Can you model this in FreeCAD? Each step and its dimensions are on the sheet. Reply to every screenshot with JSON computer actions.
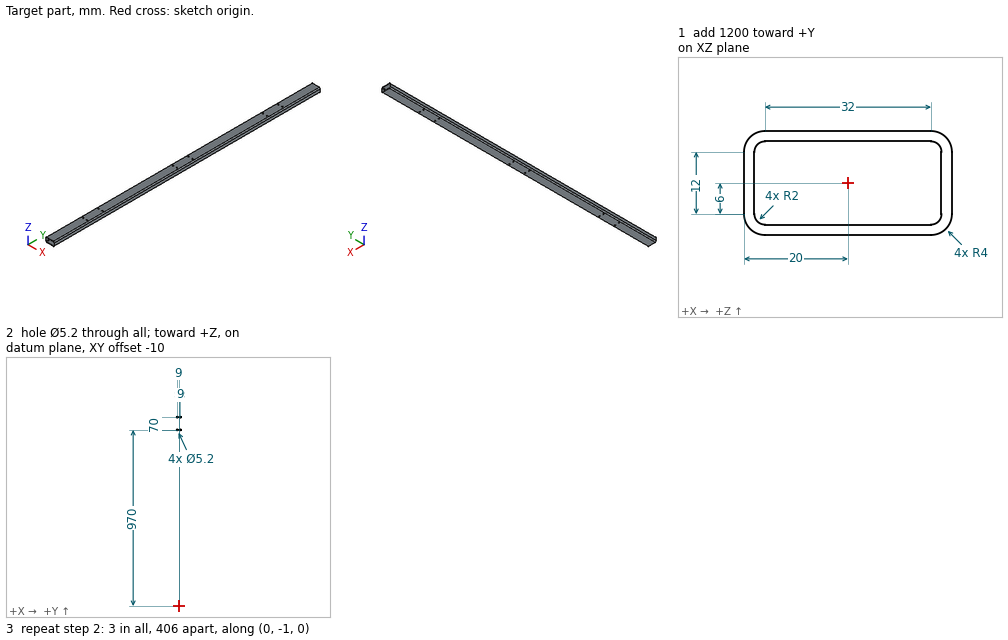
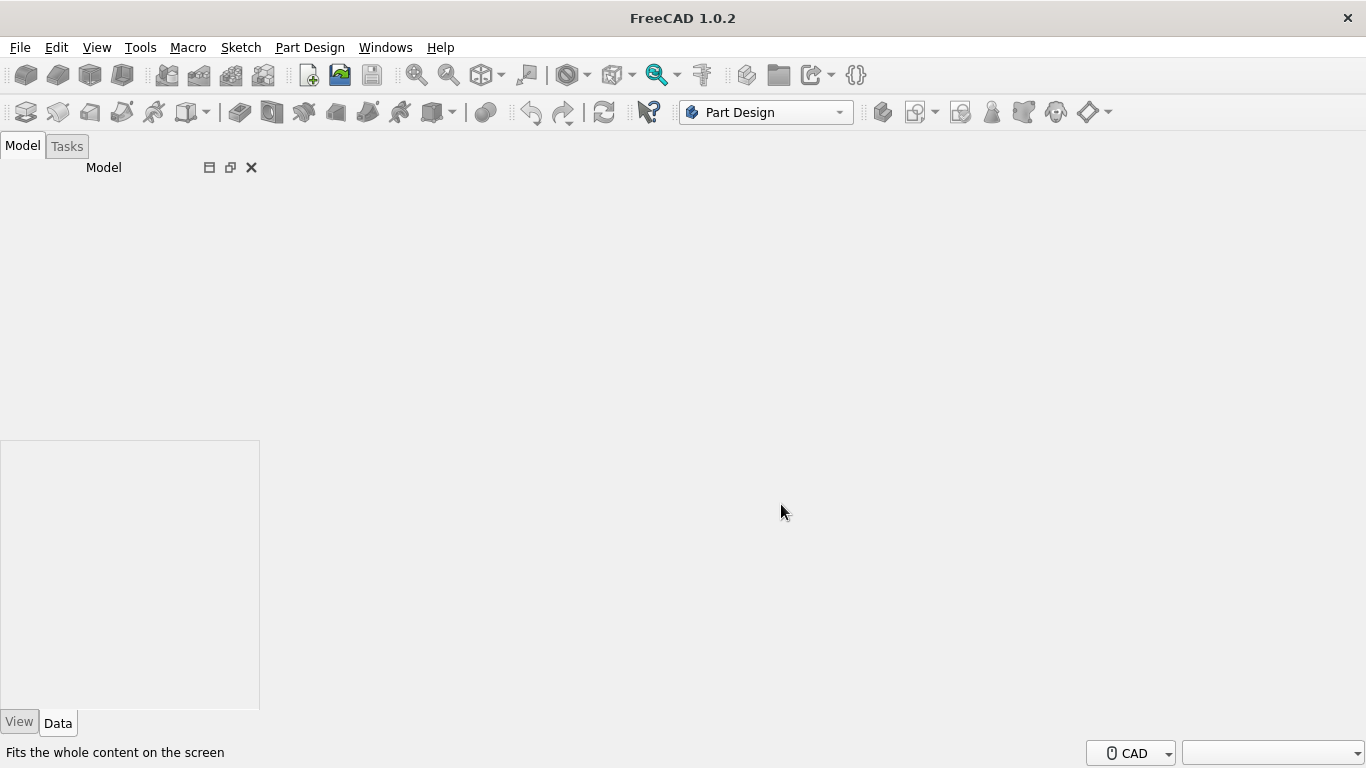
{"action": "left_click", "coordinate": [308, 76]}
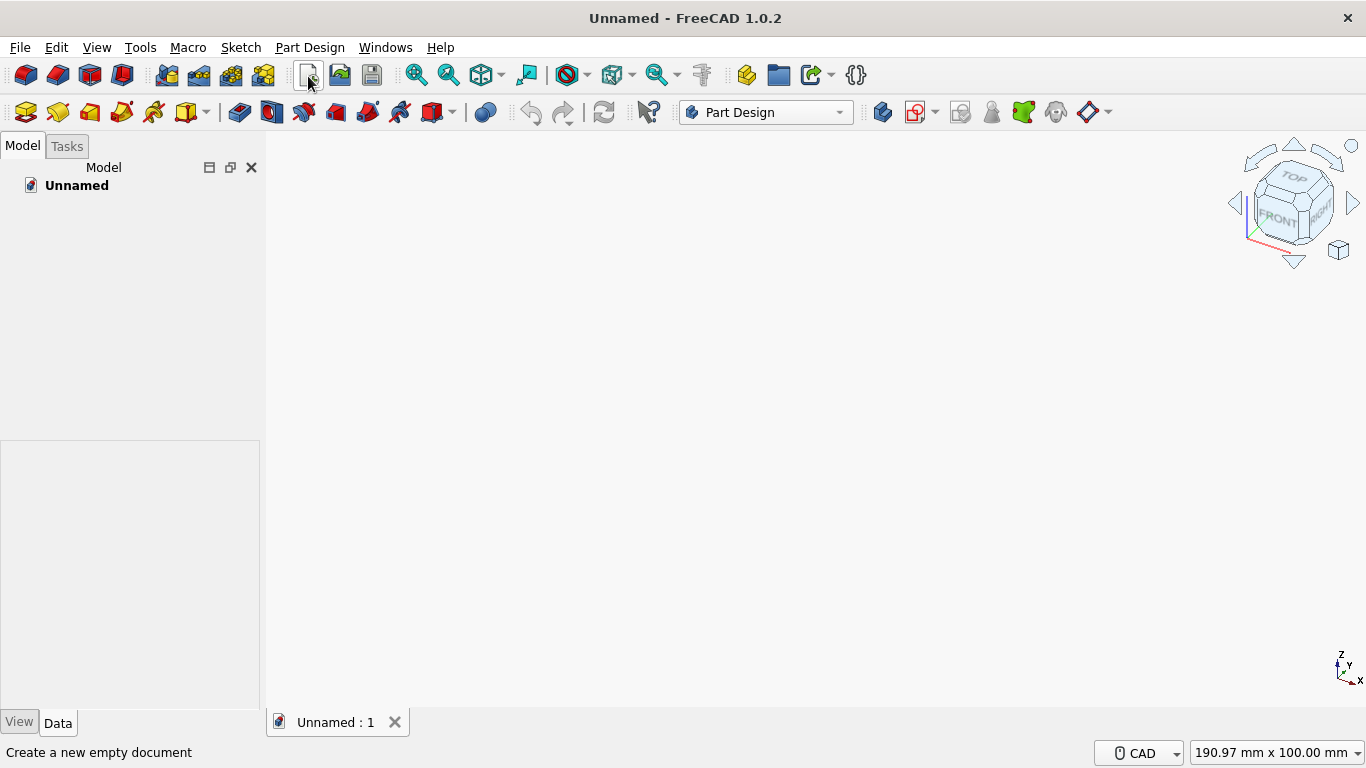
{"action": "left_click", "coordinate": [916, 112]}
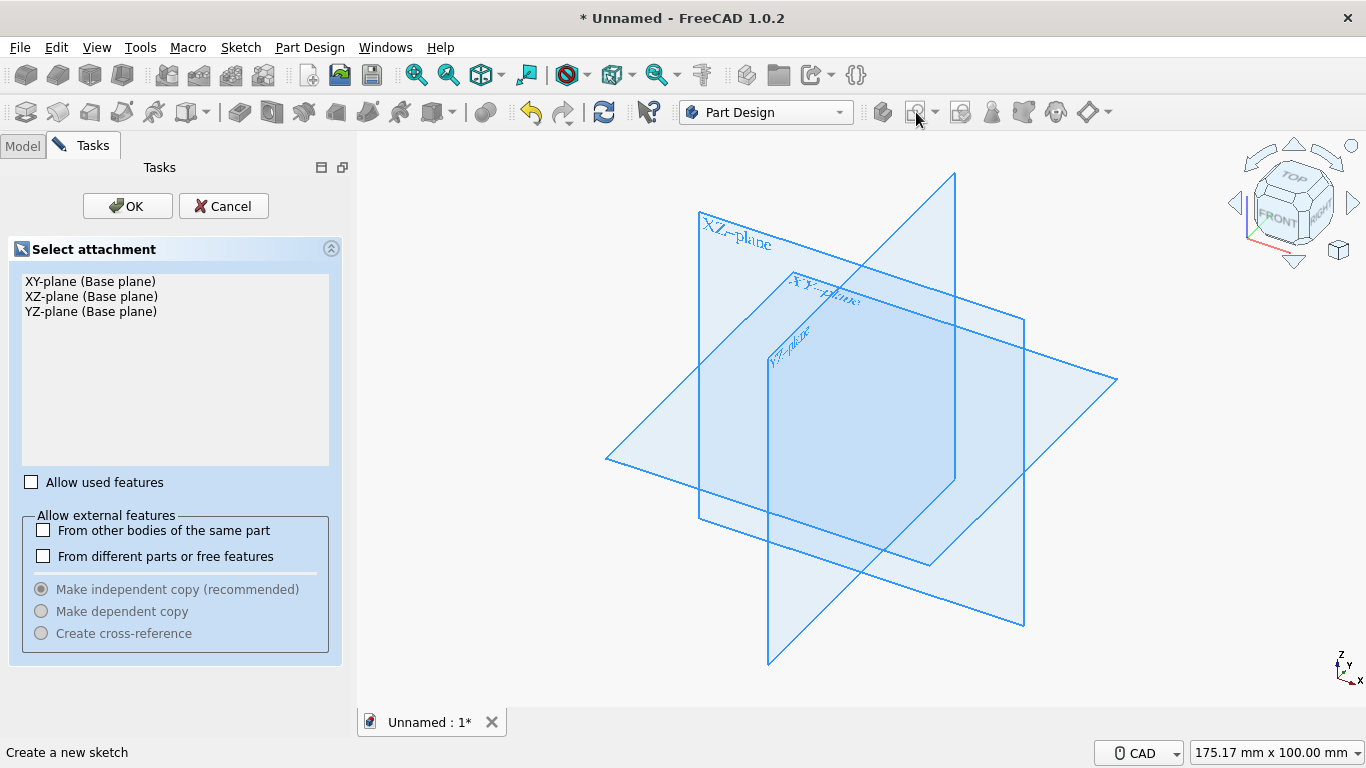
{"action": "left_click", "coordinate": [82, 296]}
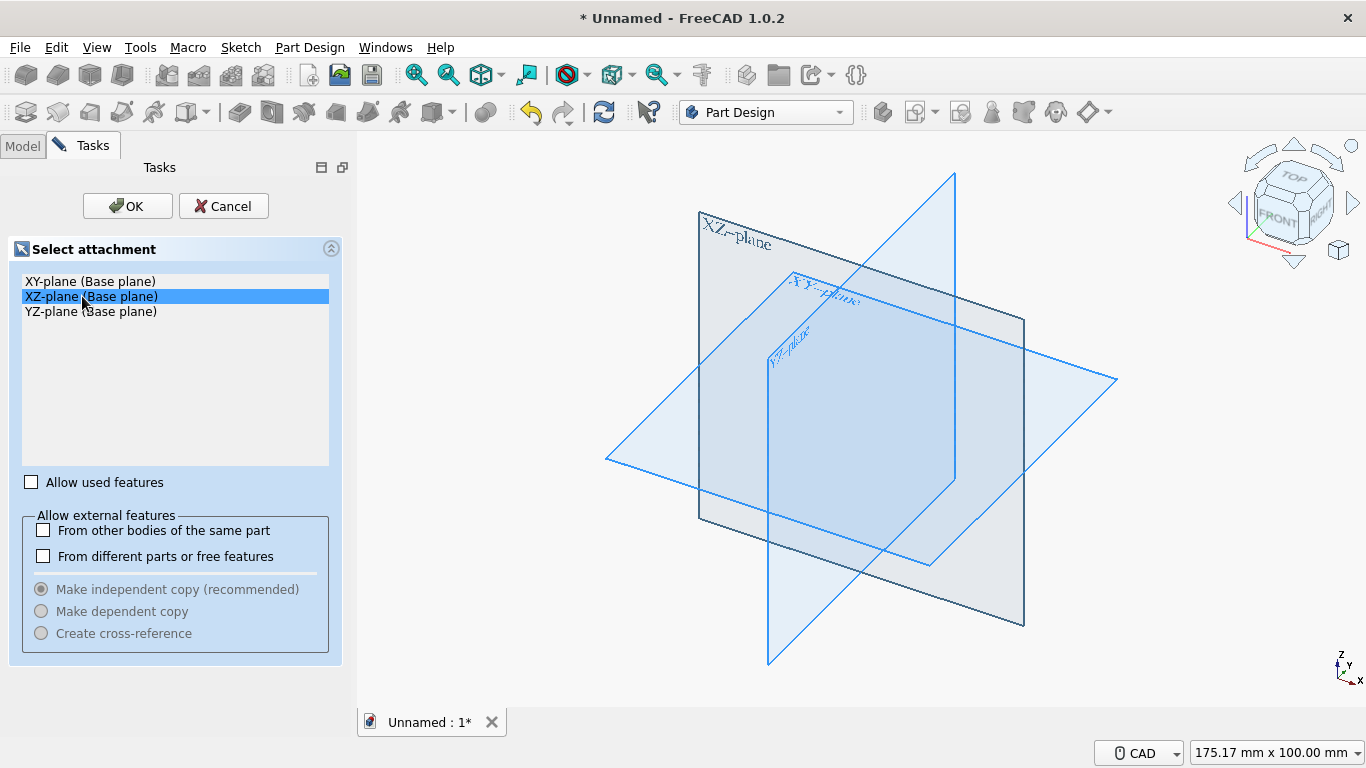
{"action": "left_click", "coordinate": [128, 206]}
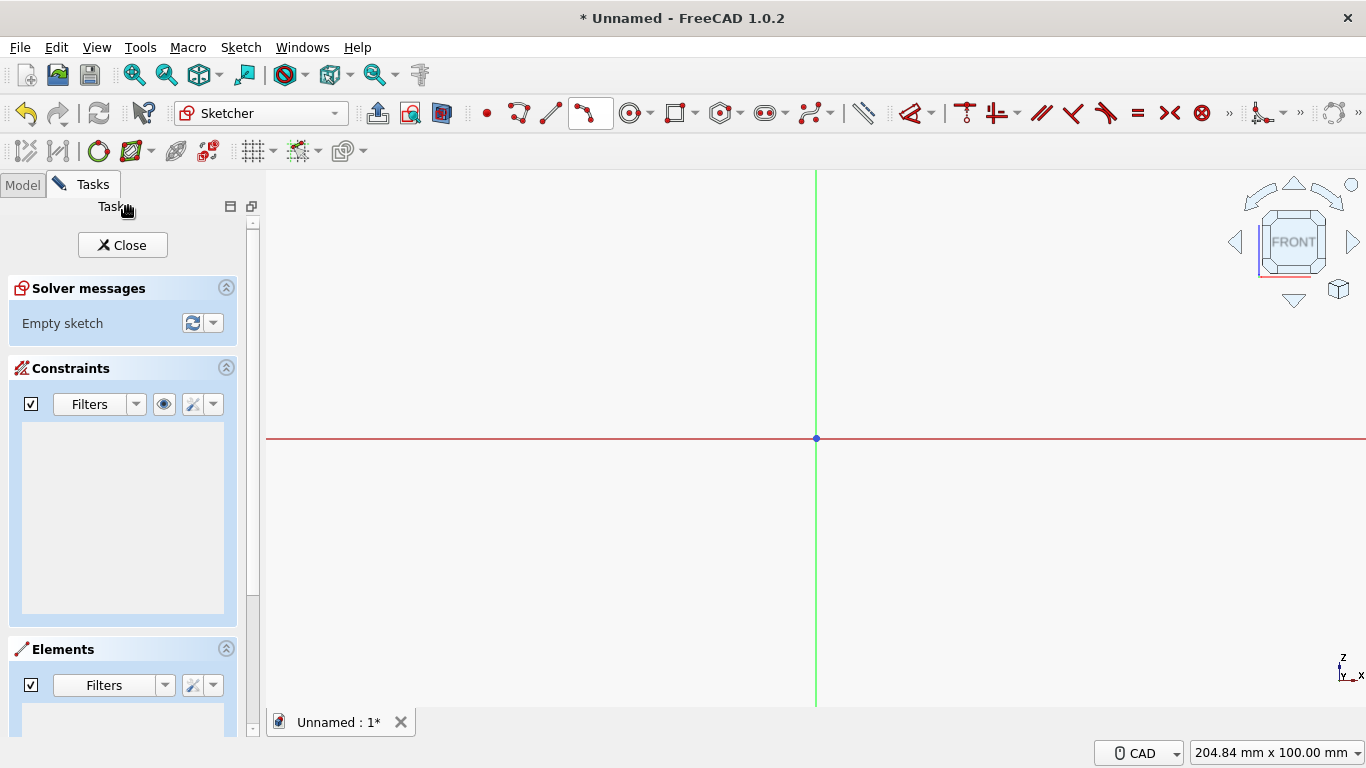
{"action": "scroll", "coordinate": [856, 439], "scroll_direction": "up", "scroll_amount": 5}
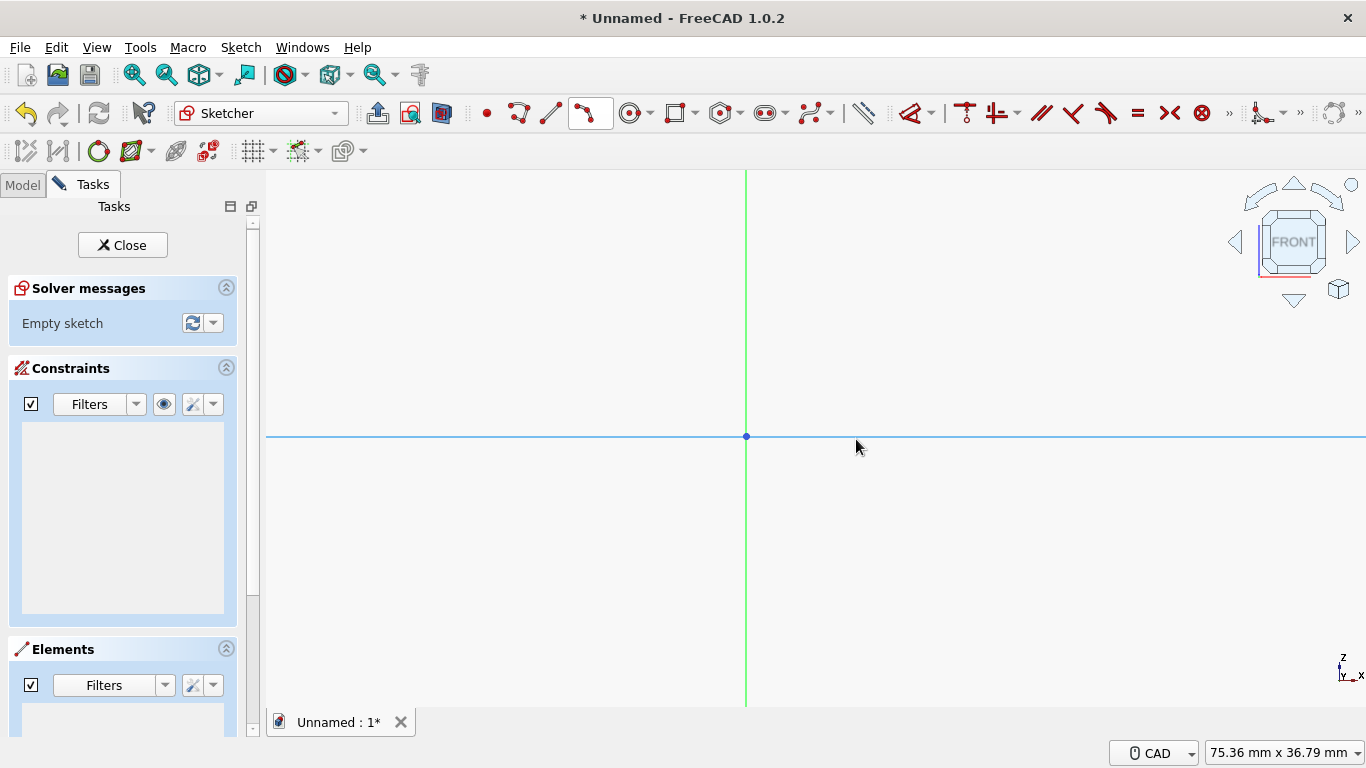
{"action": "left_click", "coordinate": [552, 114]}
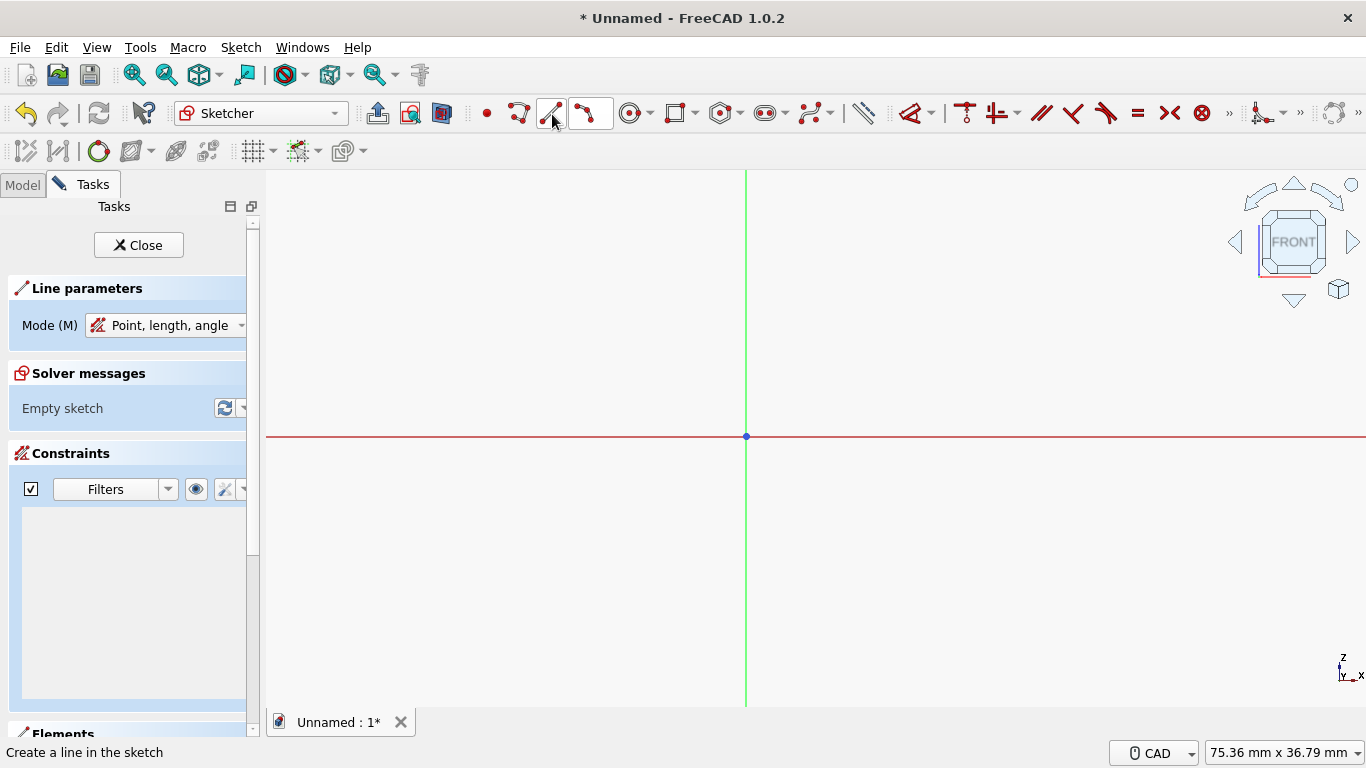
{"action": "left_click", "coordinate": [454, 524]}
{"action": "left_click", "coordinate": [454, 349]}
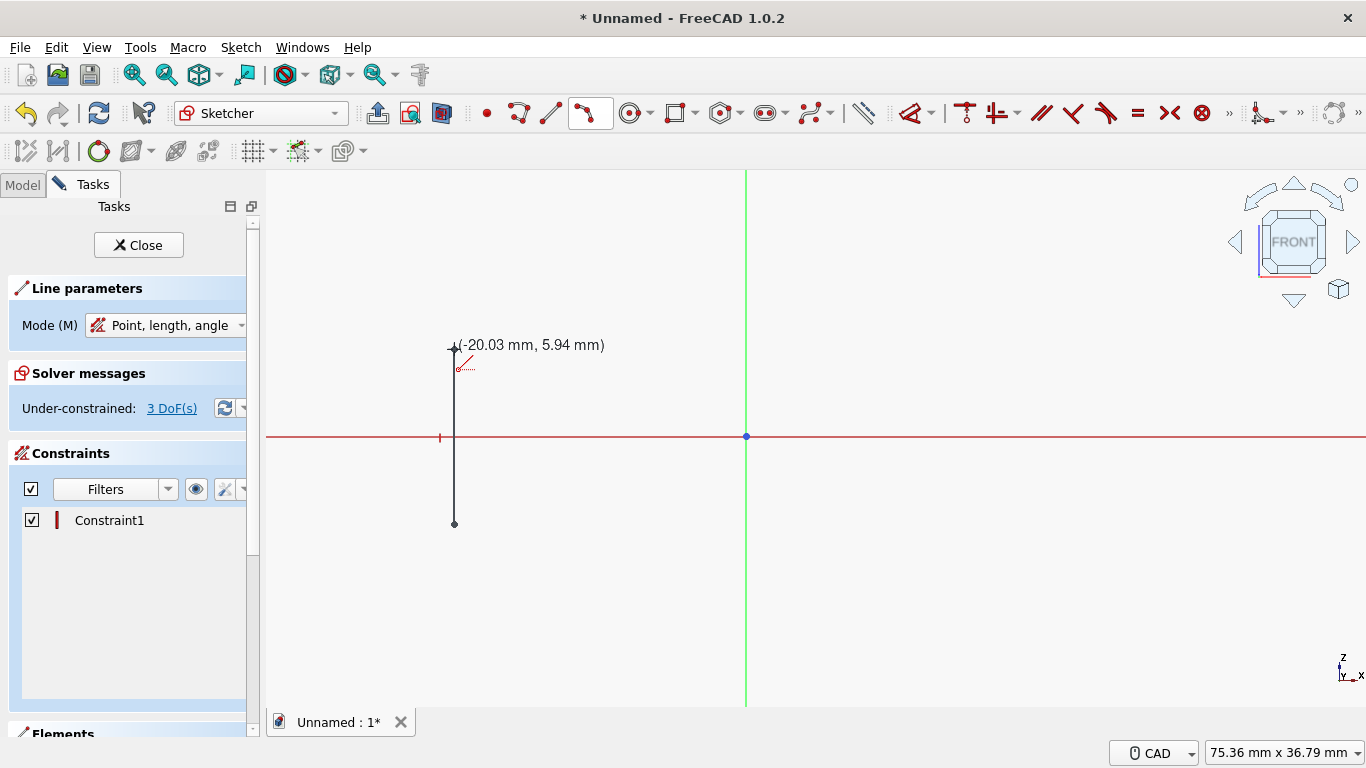
{"action": "left_click", "coordinate": [513, 291]}
{"action": "left_click", "coordinate": [980, 291]}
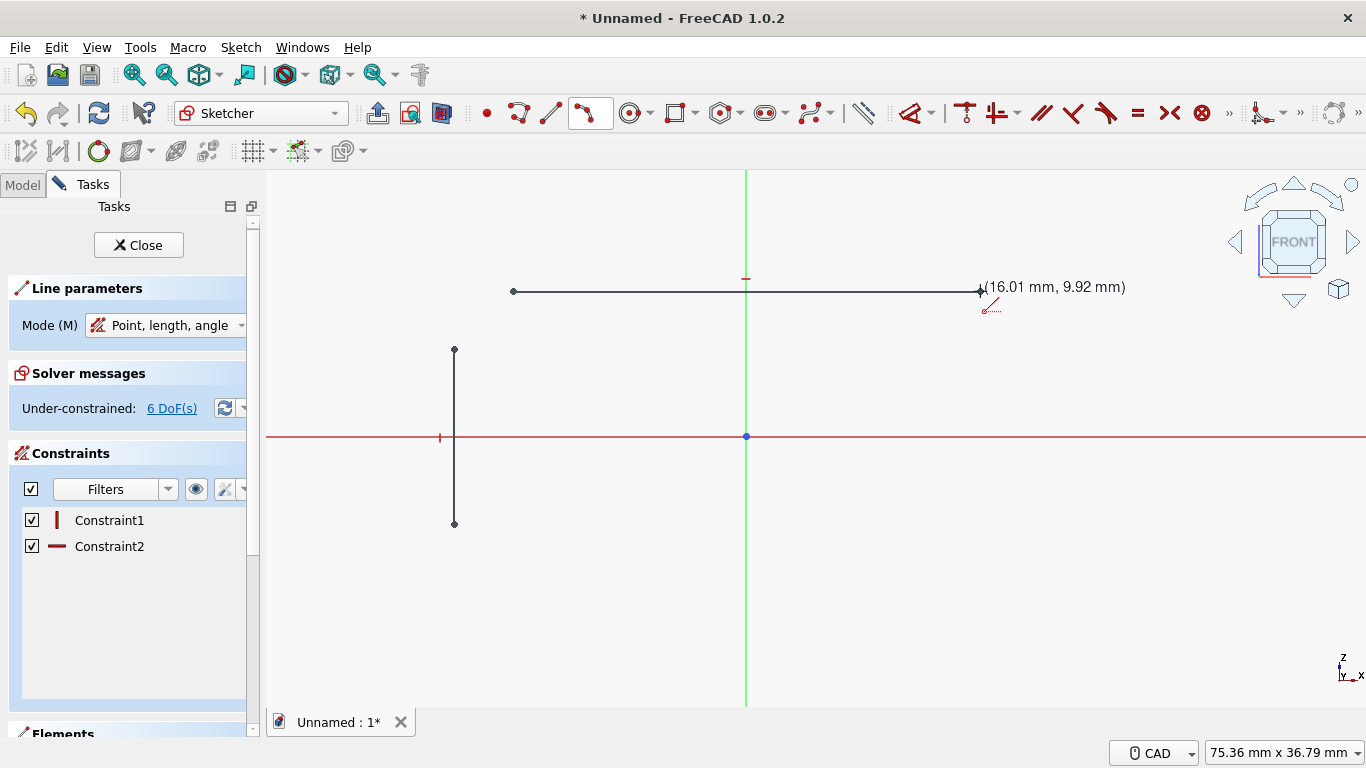
{"action": "left_click", "coordinate": [1038, 349]}
{"action": "left_click", "coordinate": [1038, 524]}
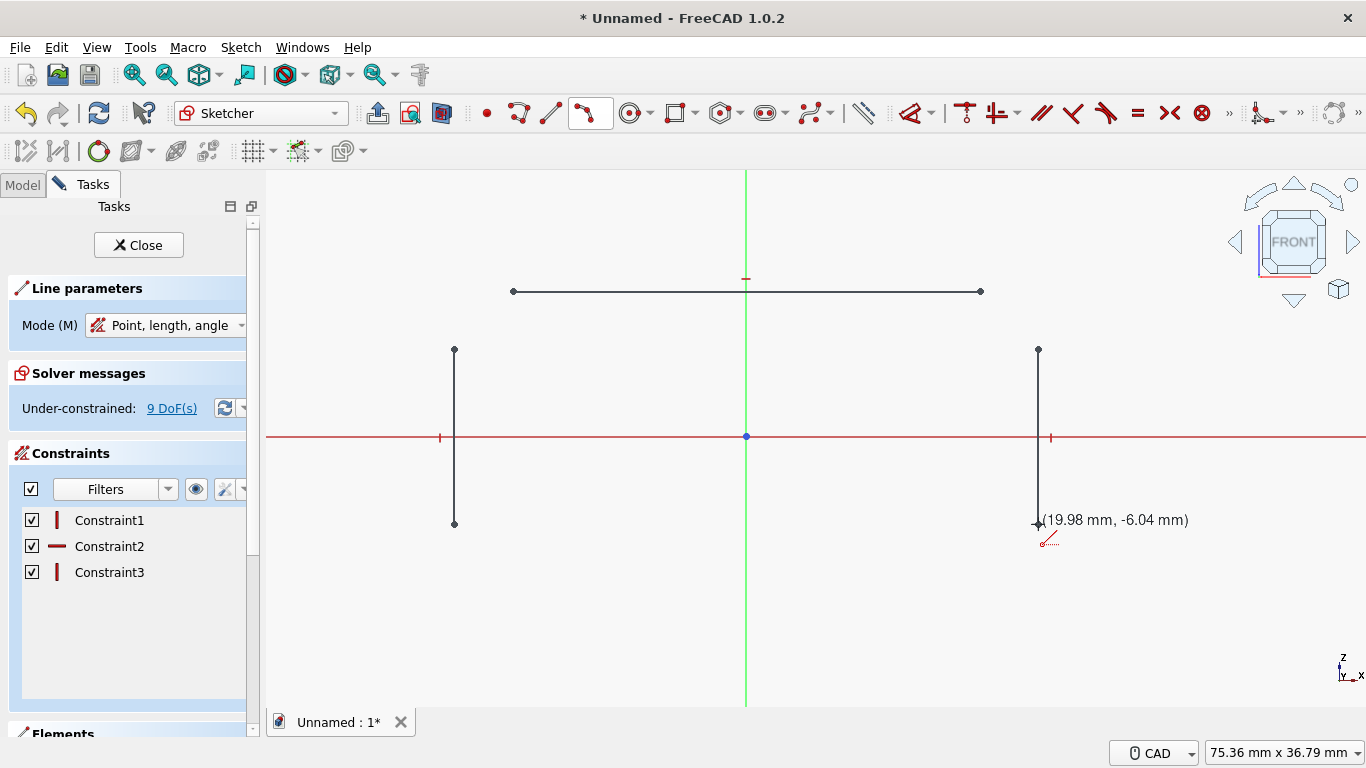
{"action": "left_click", "coordinate": [980, 583]}
{"action": "left_click", "coordinate": [513, 583]}